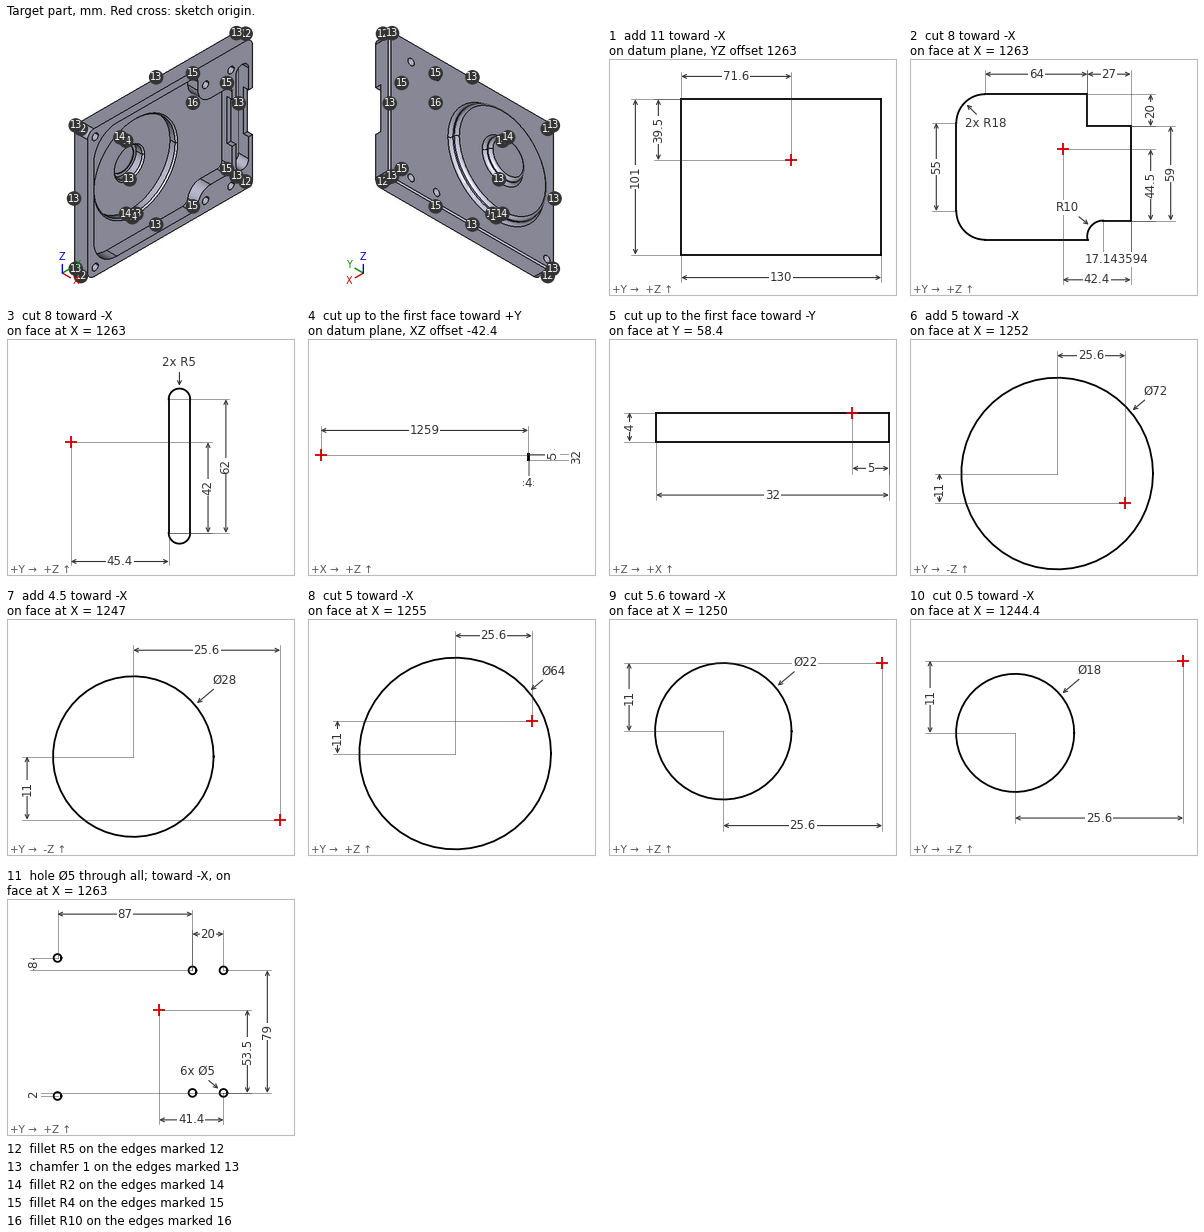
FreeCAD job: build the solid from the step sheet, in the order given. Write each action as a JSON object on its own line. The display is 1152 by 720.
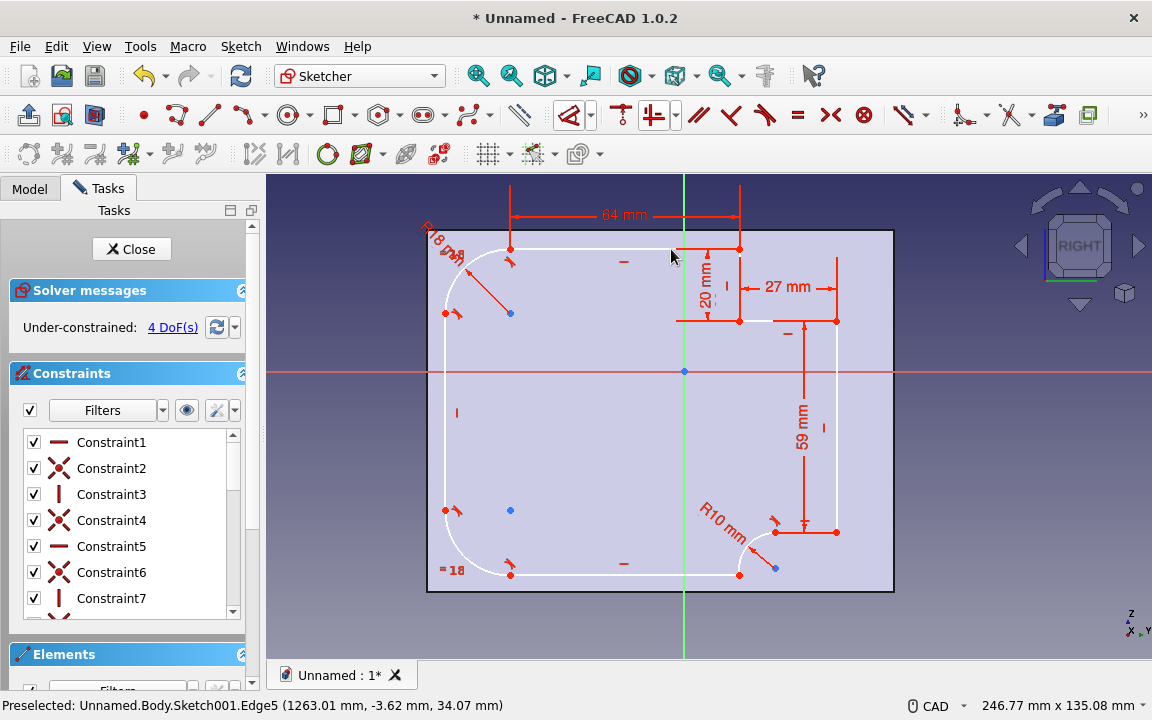
{"action": "left_click", "coordinate": [445, 373]}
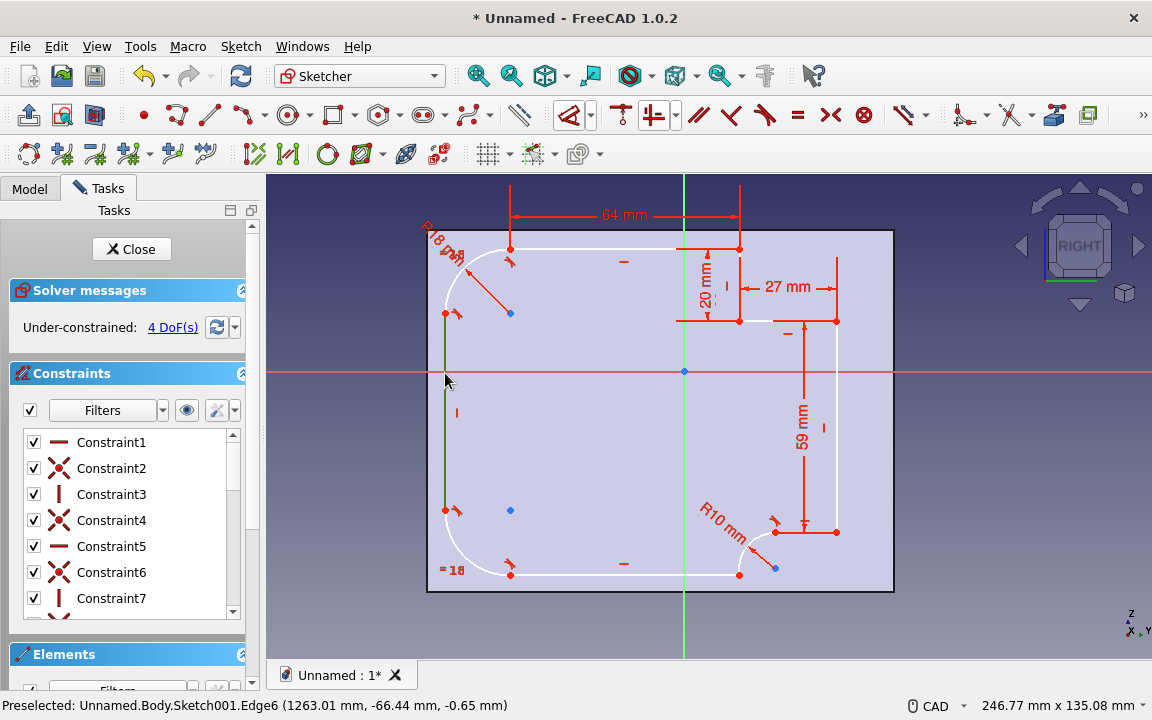
{"action": "left_click", "coordinate": [590, 116]}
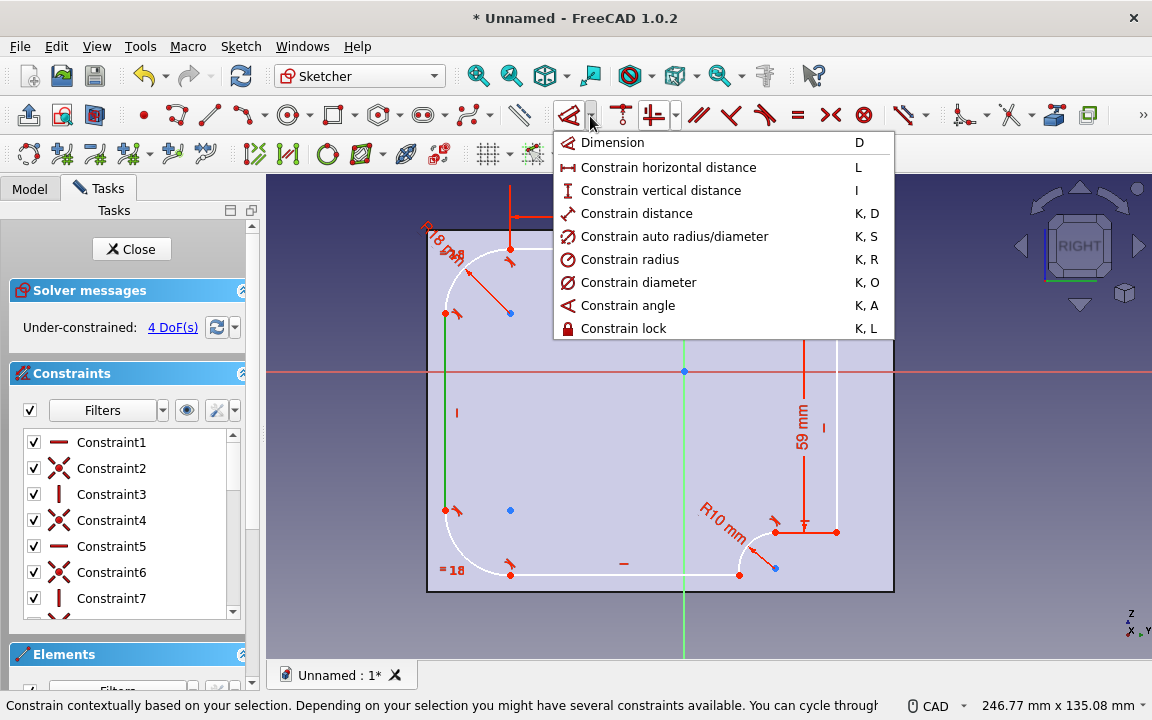
{"action": "left_click", "coordinate": [724, 190]}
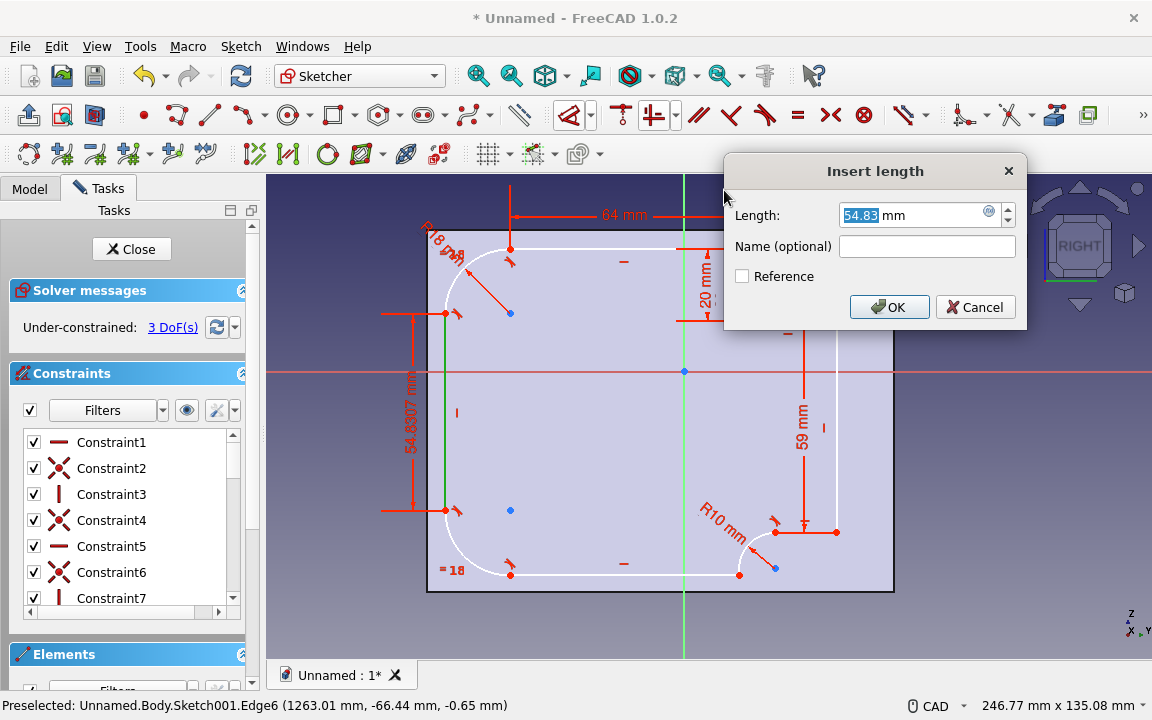
{"action": "type", "text": "55"}
{"action": "key", "text": "Return"}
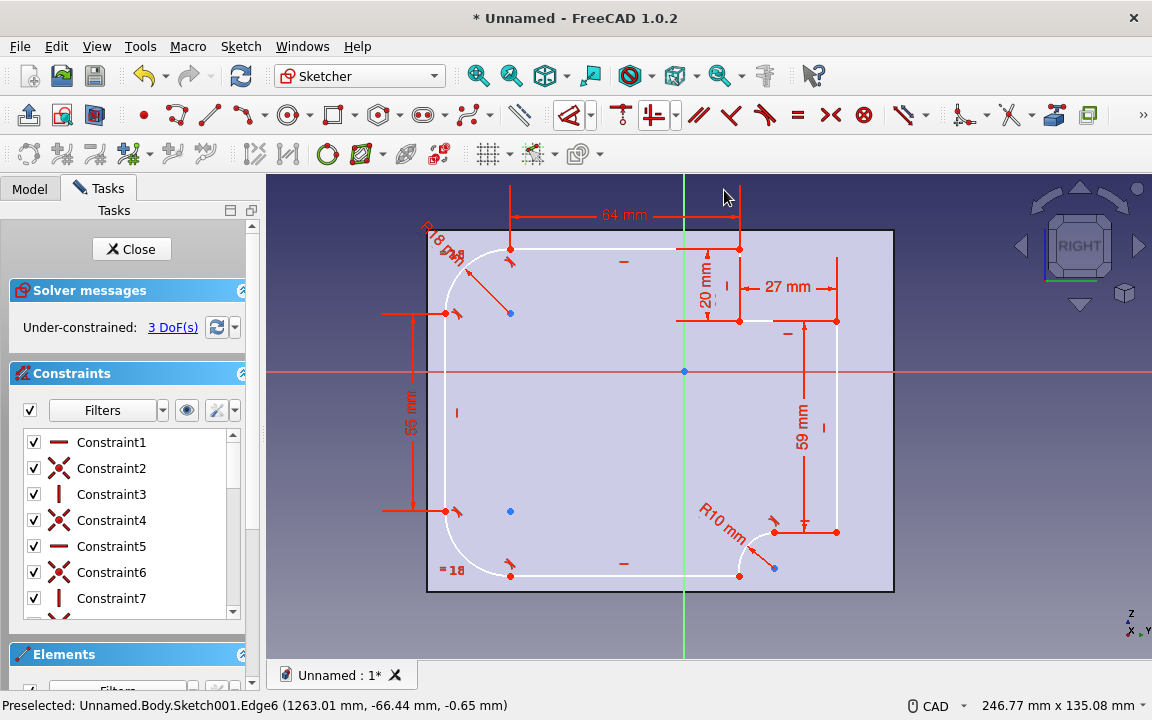
{"action": "left_click", "coordinate": [775, 533]}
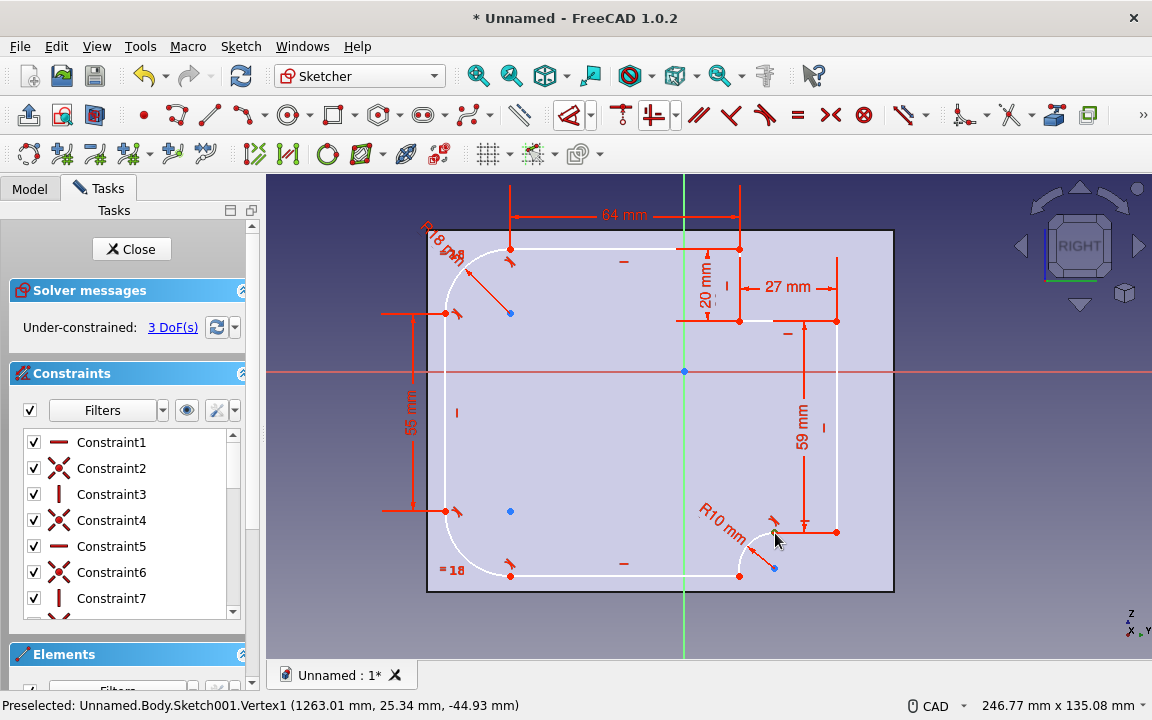
{"action": "left_click", "coordinate": [590, 116]}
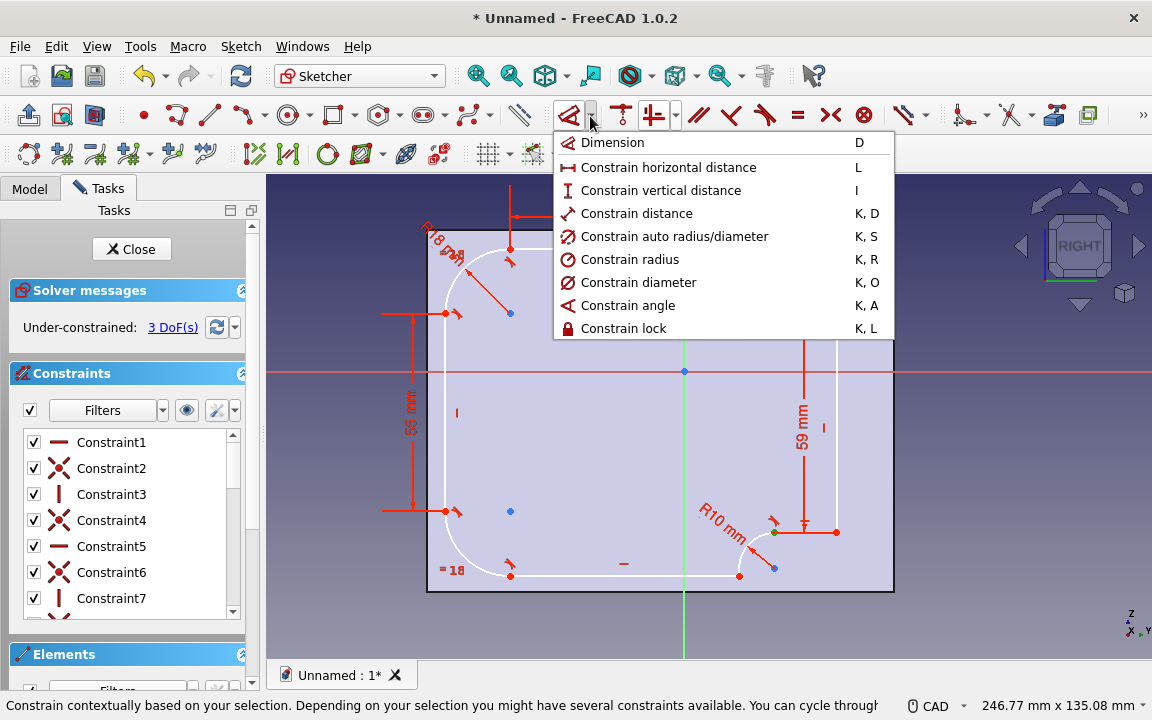
{"action": "left_click", "coordinate": [724, 190]}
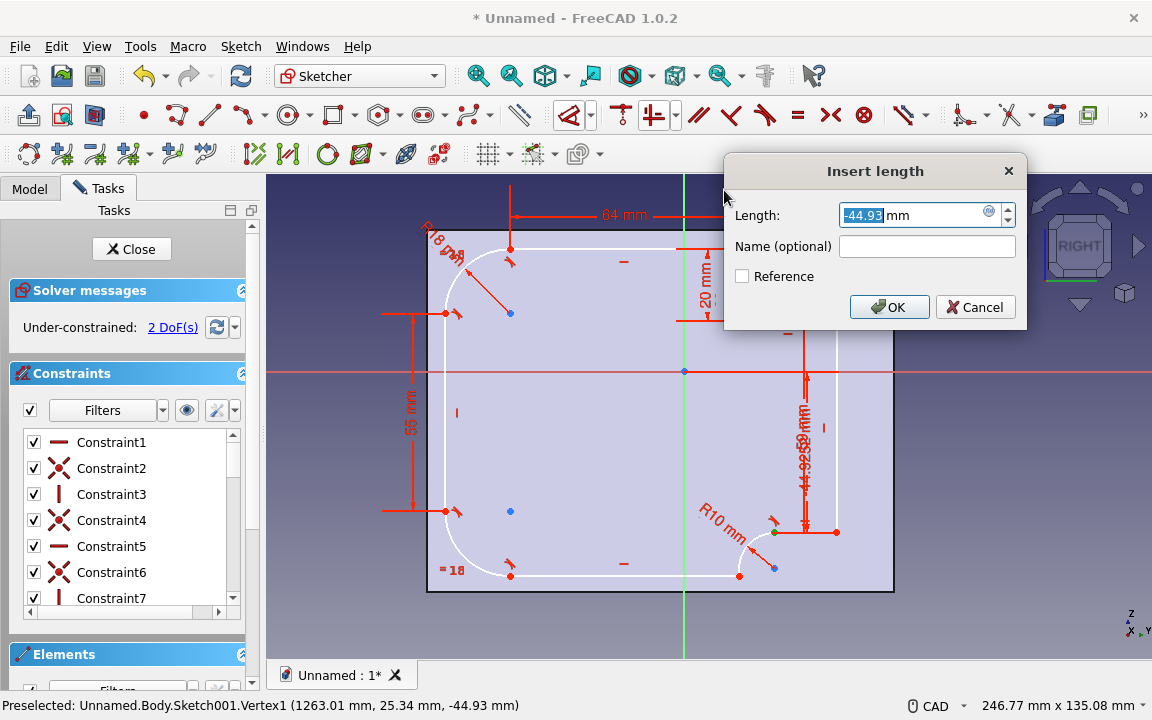
{"action": "type", "text": "-44.5"}
{"action": "key", "text": "Return"}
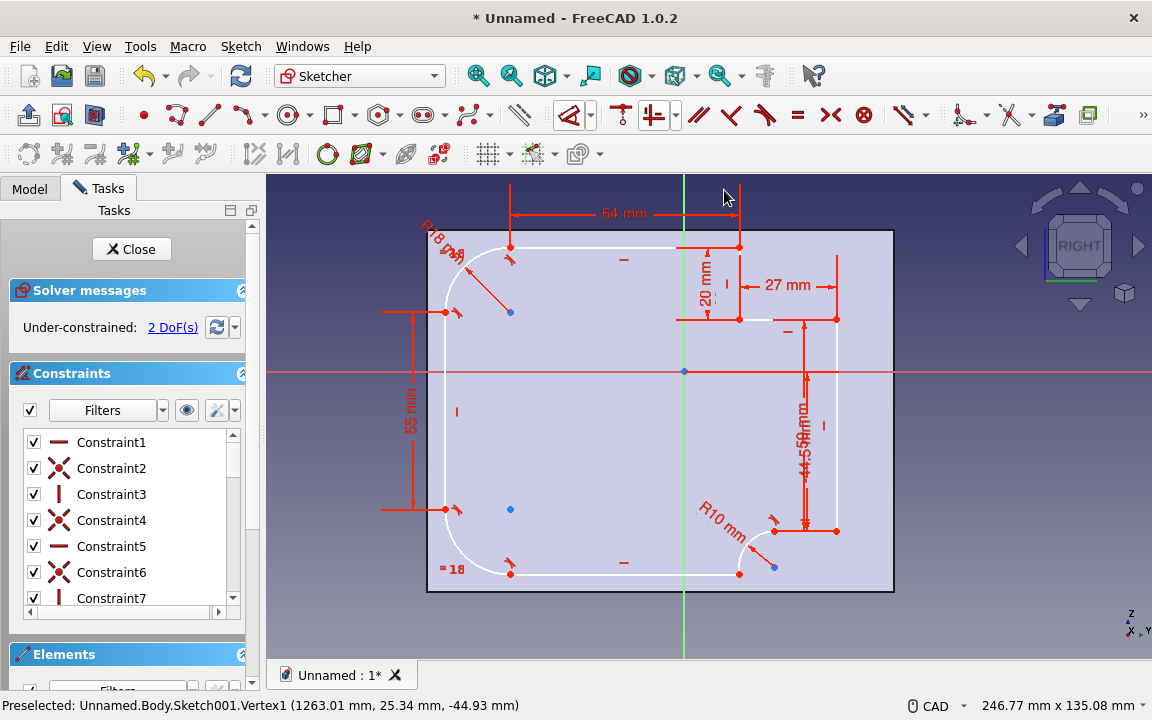
{"action": "left_click", "coordinate": [837, 531]}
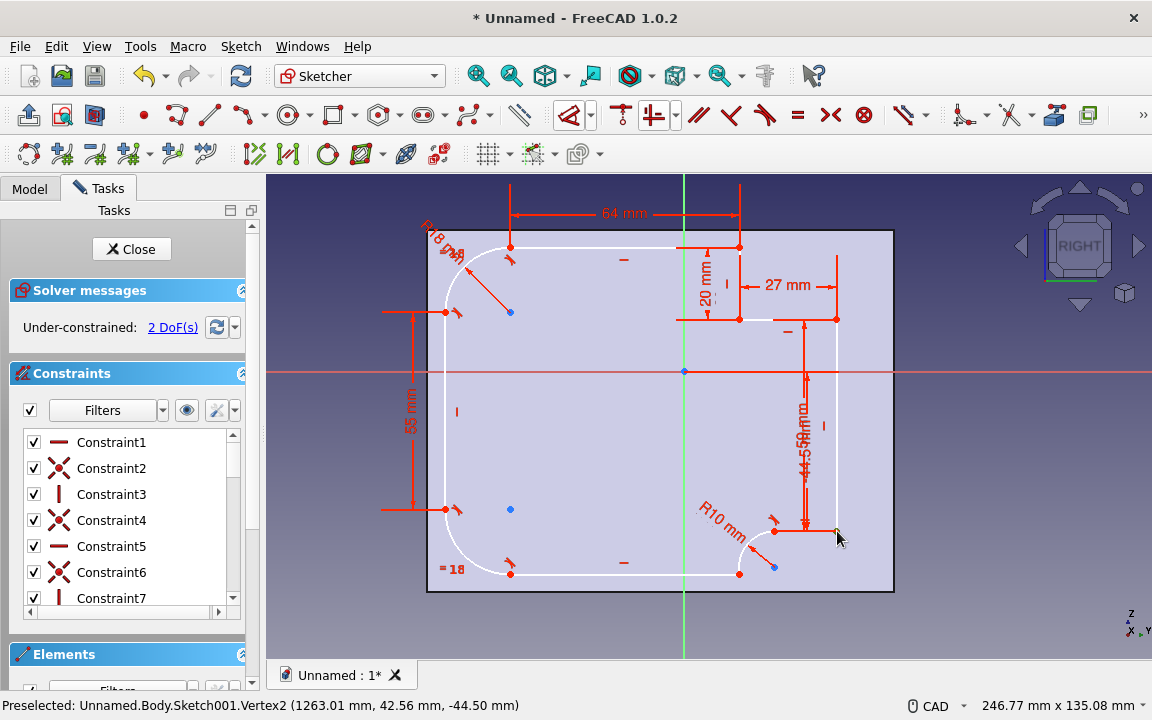
{"action": "key", "text": "l"}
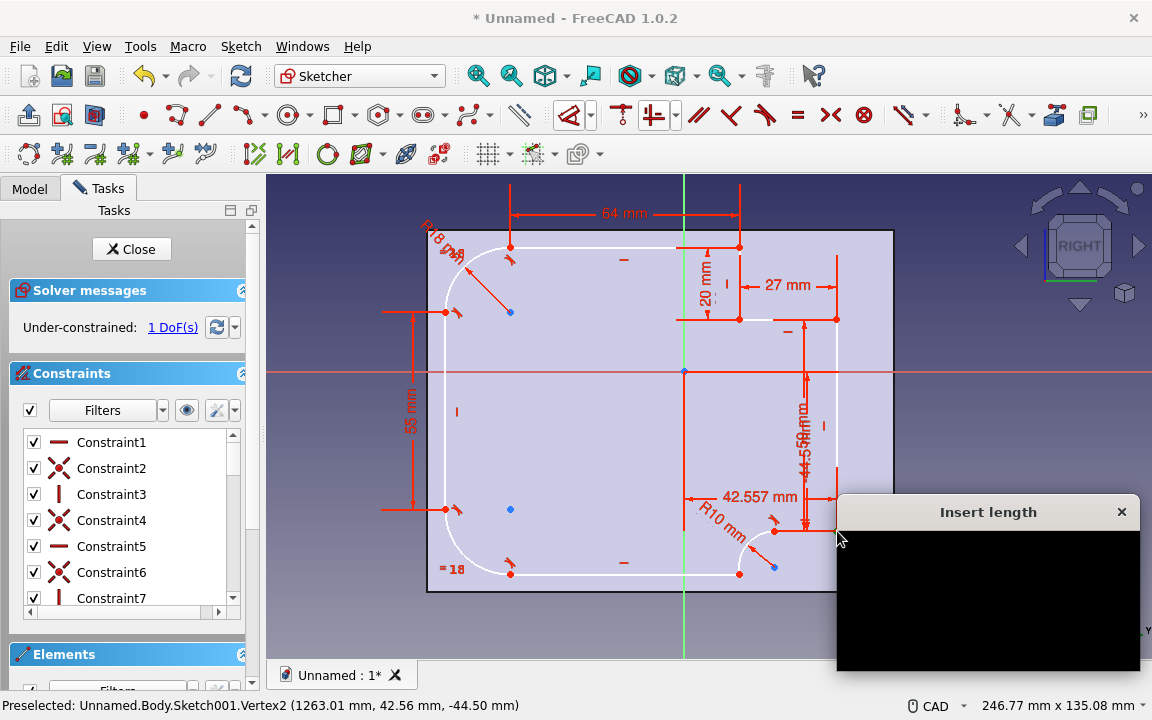
{"action": "type", "text": "42.4"}
{"action": "key", "text": "Return"}